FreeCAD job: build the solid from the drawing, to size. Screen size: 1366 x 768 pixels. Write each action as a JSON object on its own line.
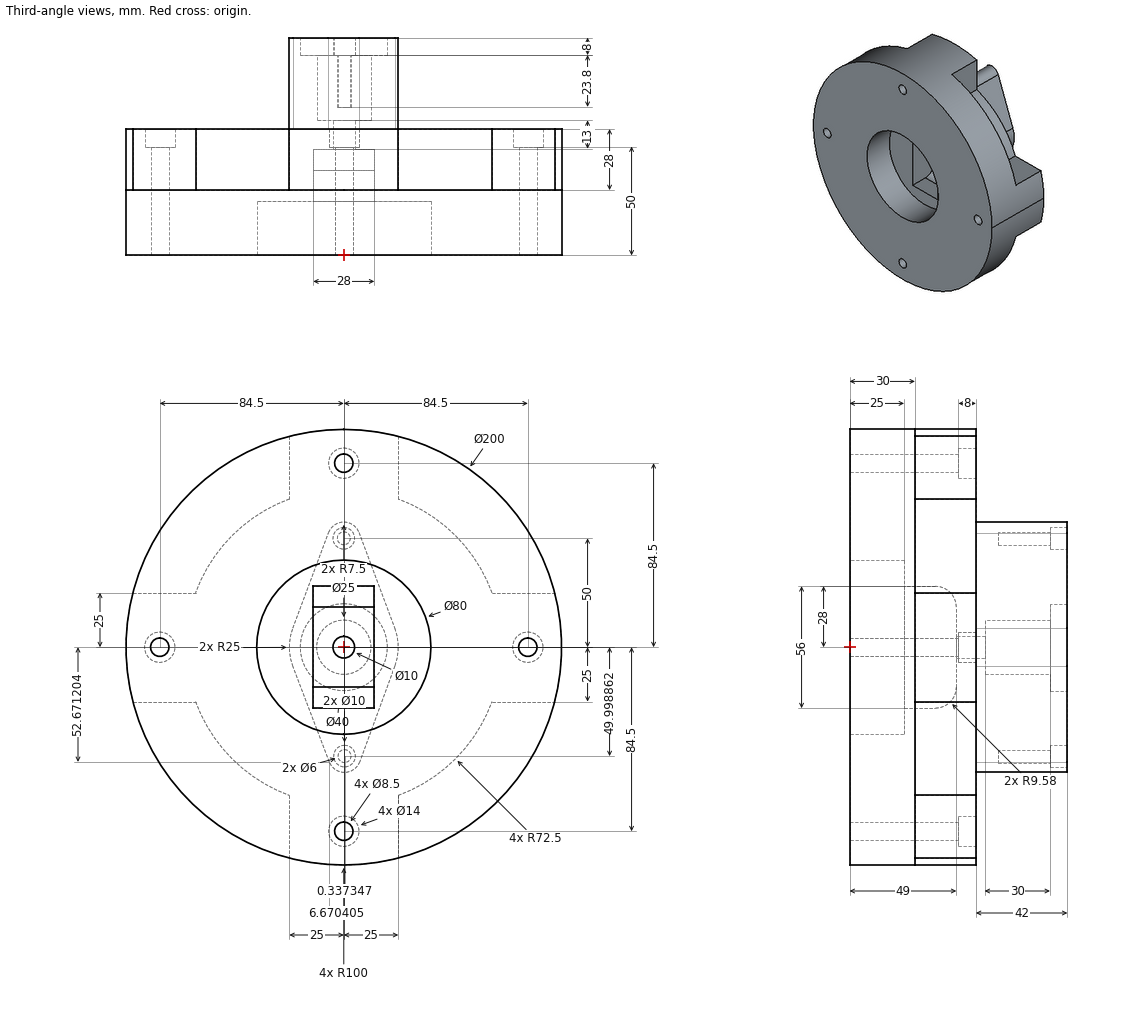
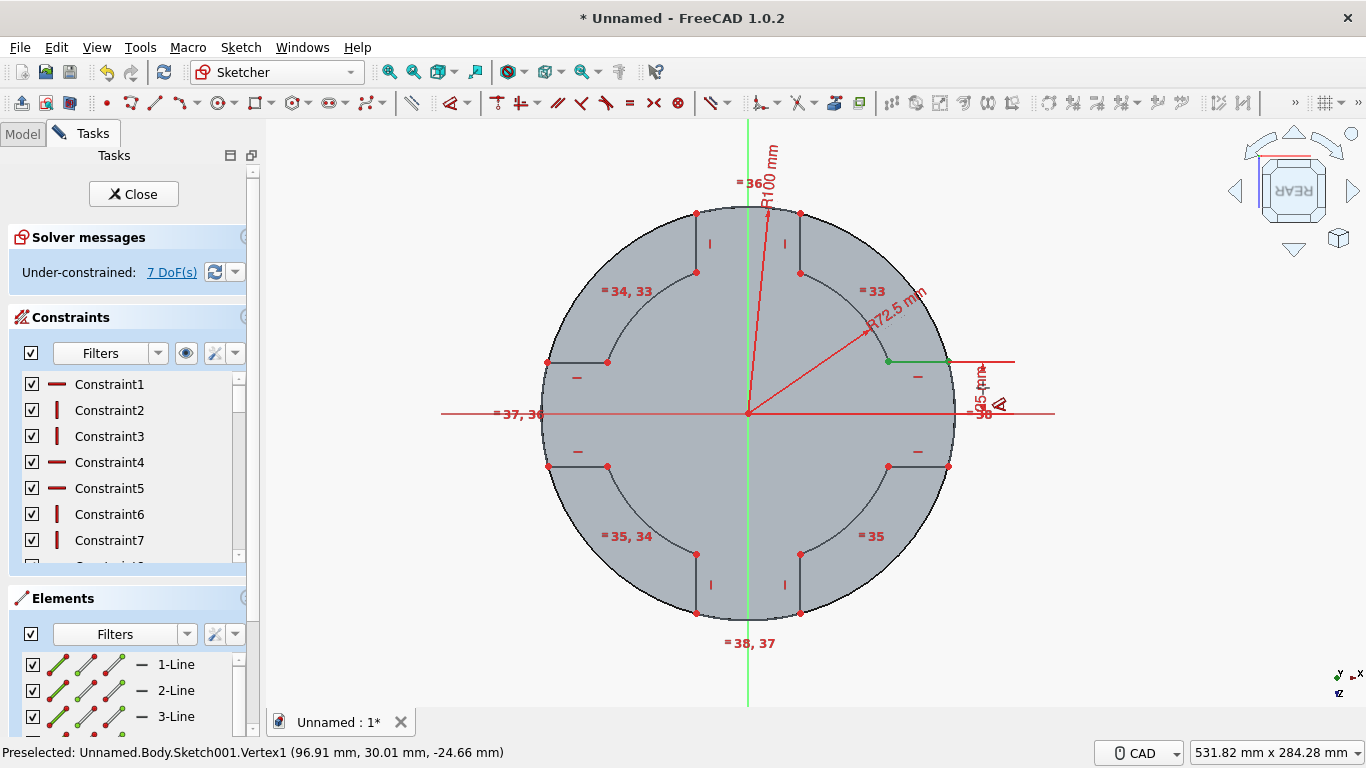
{"action": "left_click", "coordinate": [800, 273]}
{"action": "left_click", "coordinate": [774, 239]}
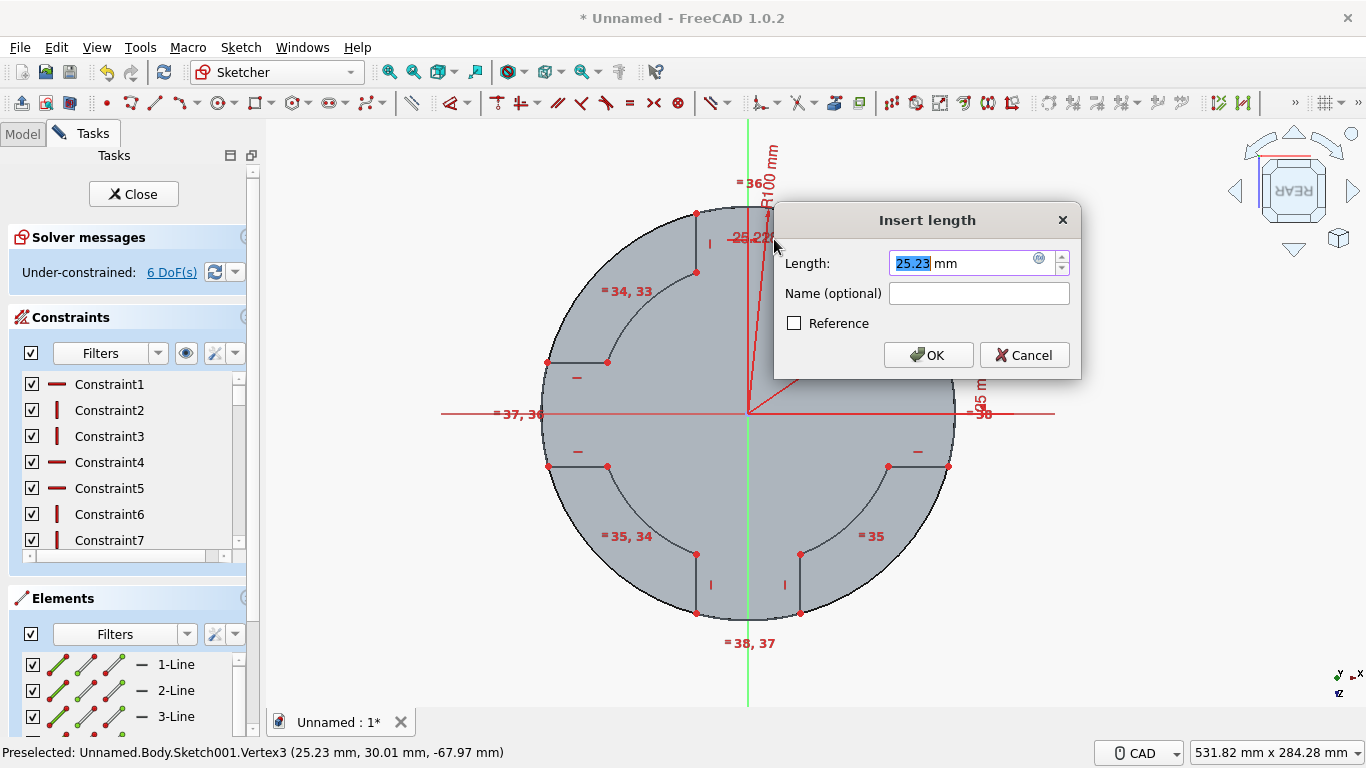
{"action": "type", "text": "25"}
{"action": "key", "text": "Return"}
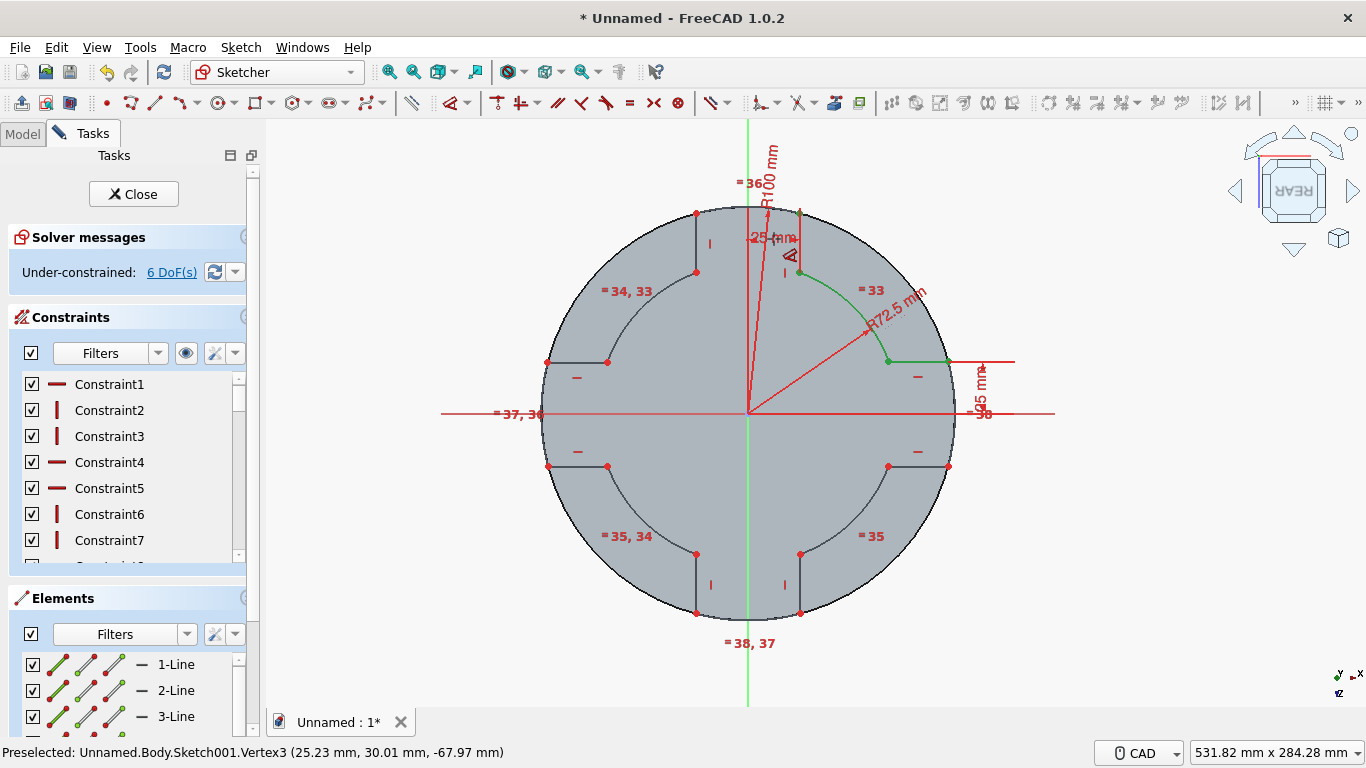
{"action": "left_click", "coordinate": [696, 213]}
{"action": "left_click", "coordinate": [722, 448]}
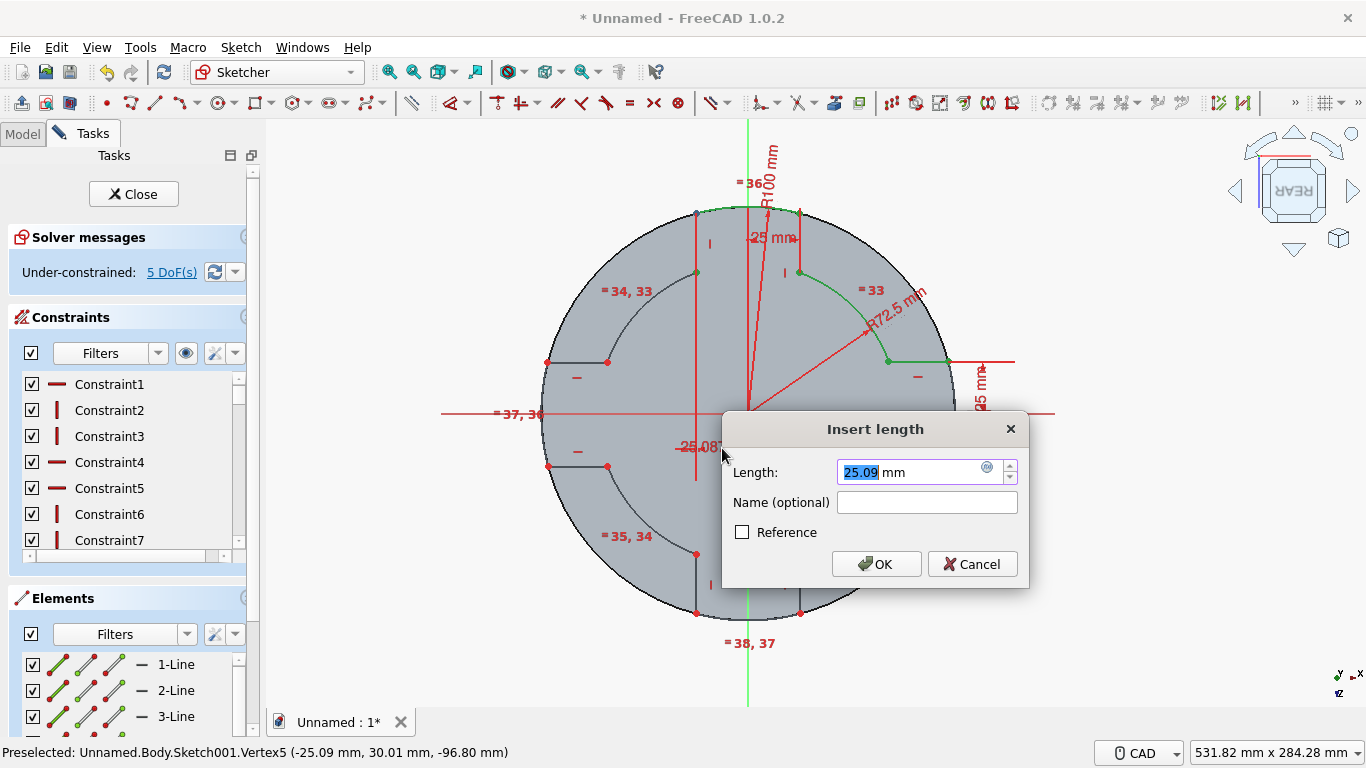
{"action": "type", "text": "25"}
{"action": "key", "text": "Return"}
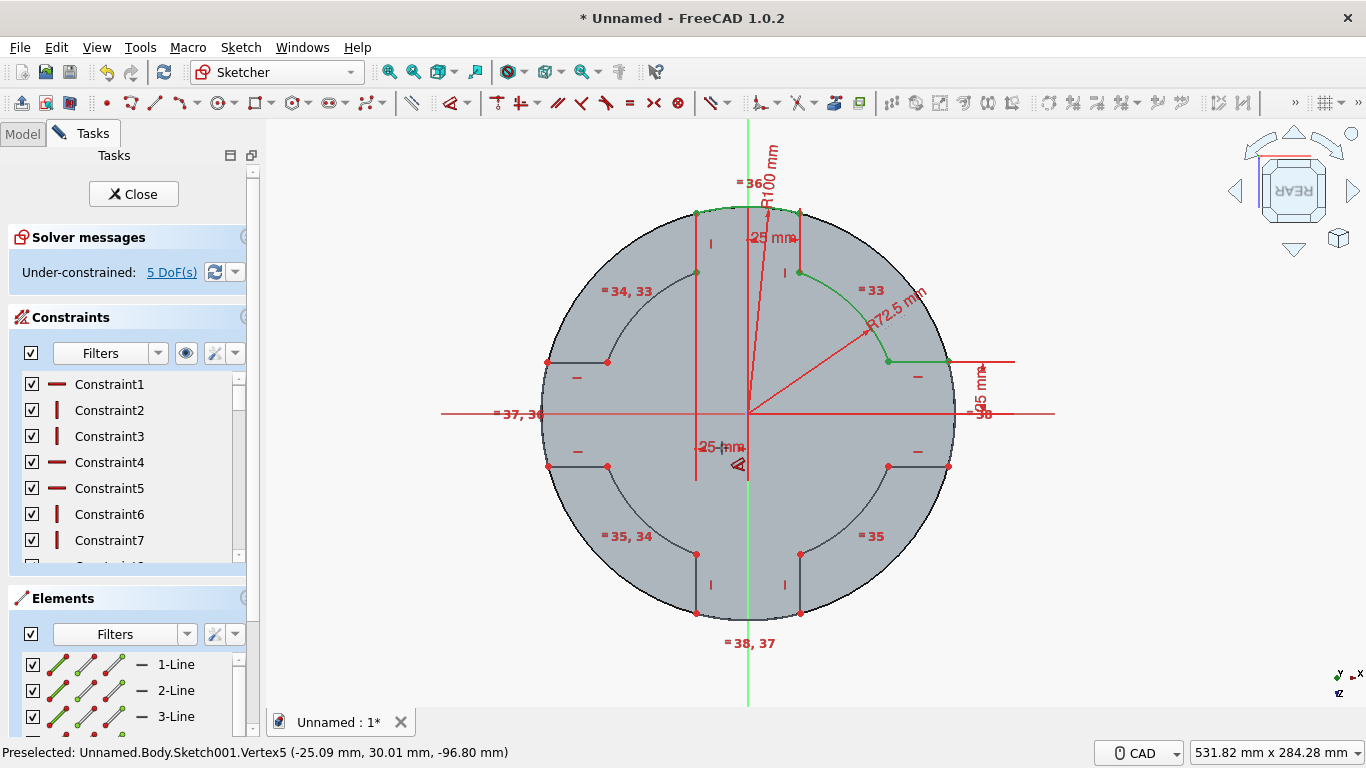
{"action": "left_click", "coordinate": [607, 363]}
{"action": "left_click", "coordinate": [573, 388]}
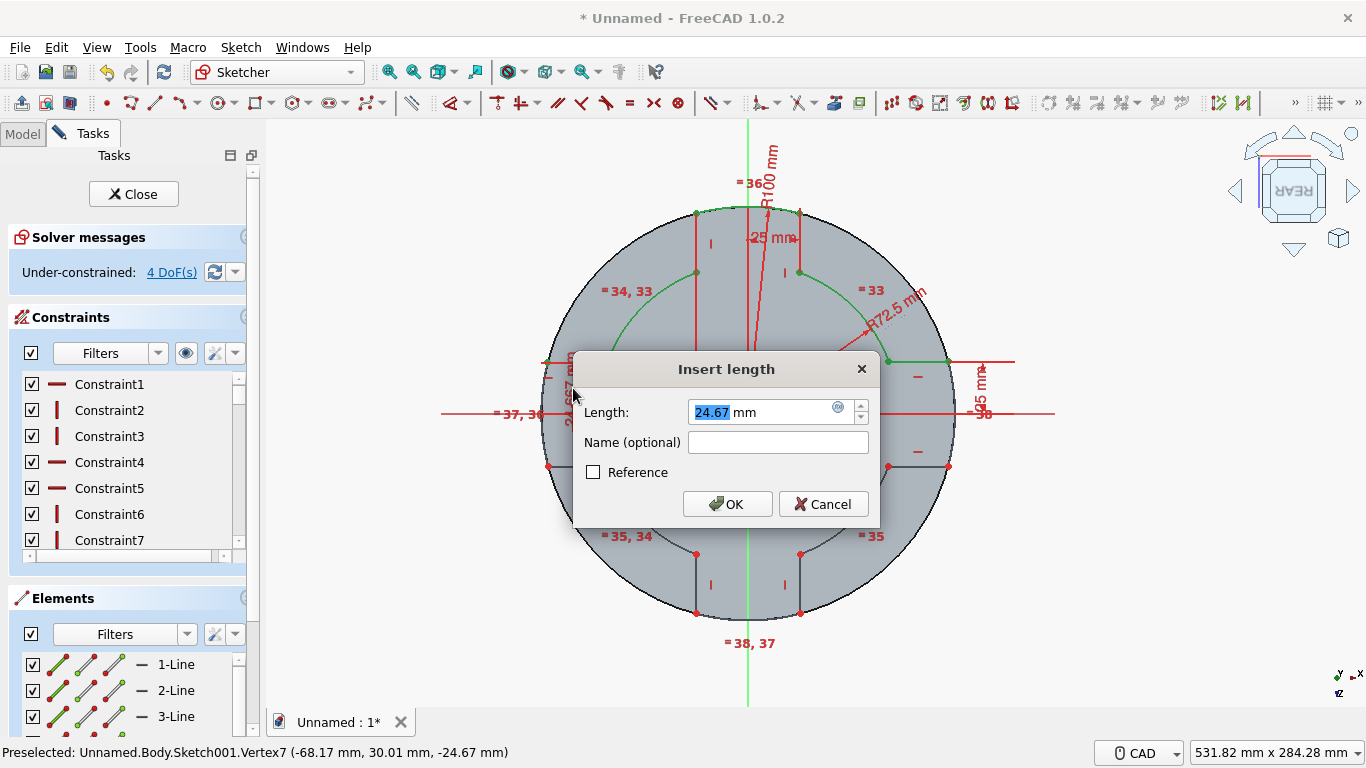
{"action": "type", "text": "25"}
{"action": "key", "text": "Return"}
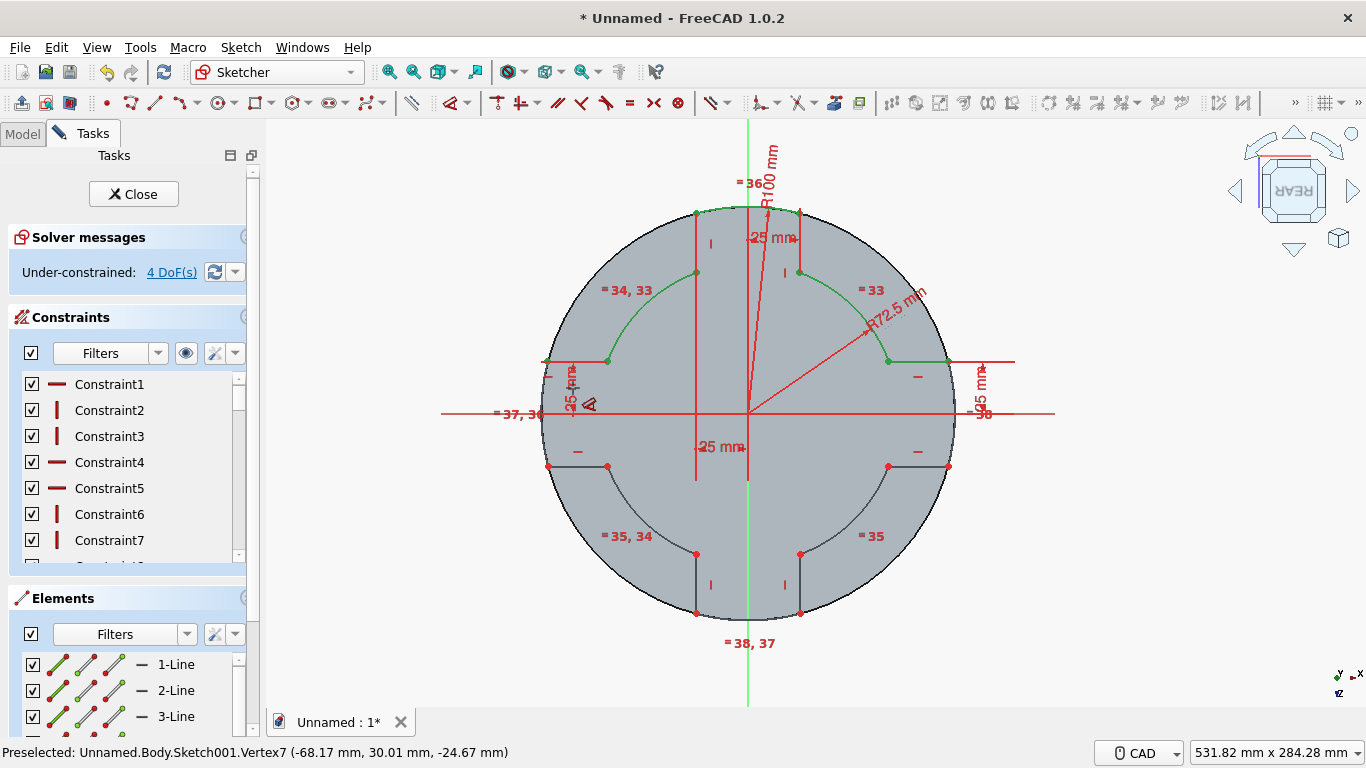
{"action": "left_click", "coordinate": [548, 467]}
{"action": "left_click", "coordinate": [514, 440]}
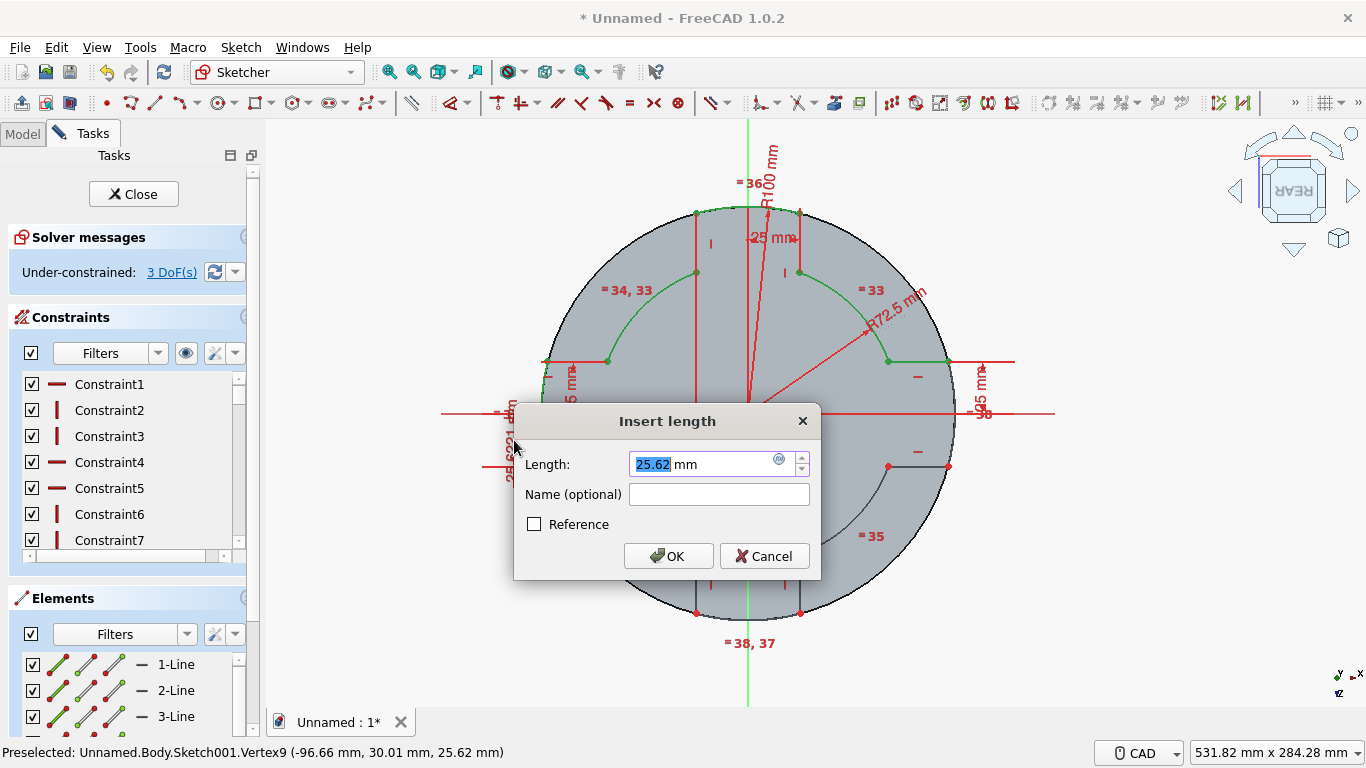
{"action": "type", "text": "25"}
{"action": "key", "text": "Return"}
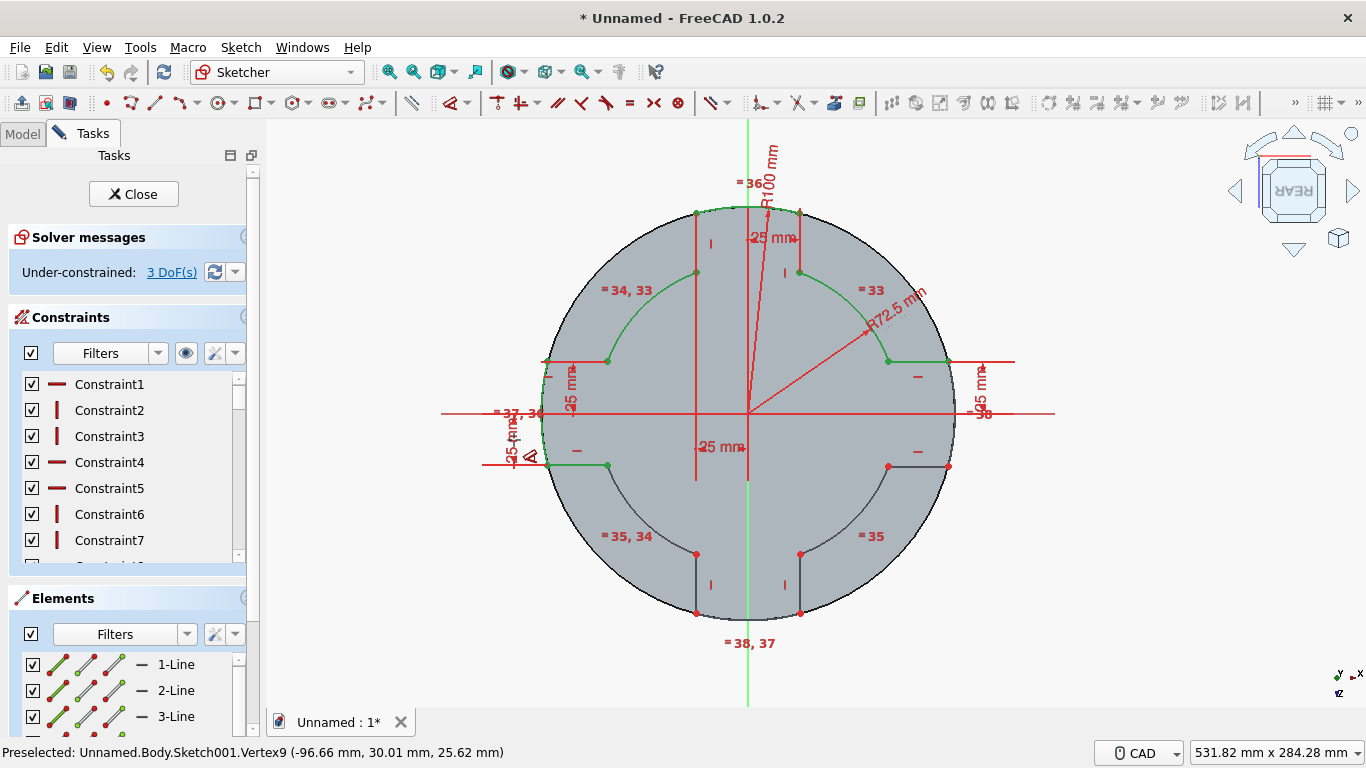
{"action": "left_click", "coordinate": [696, 554]}
{"action": "left_click", "coordinate": [722, 588]}